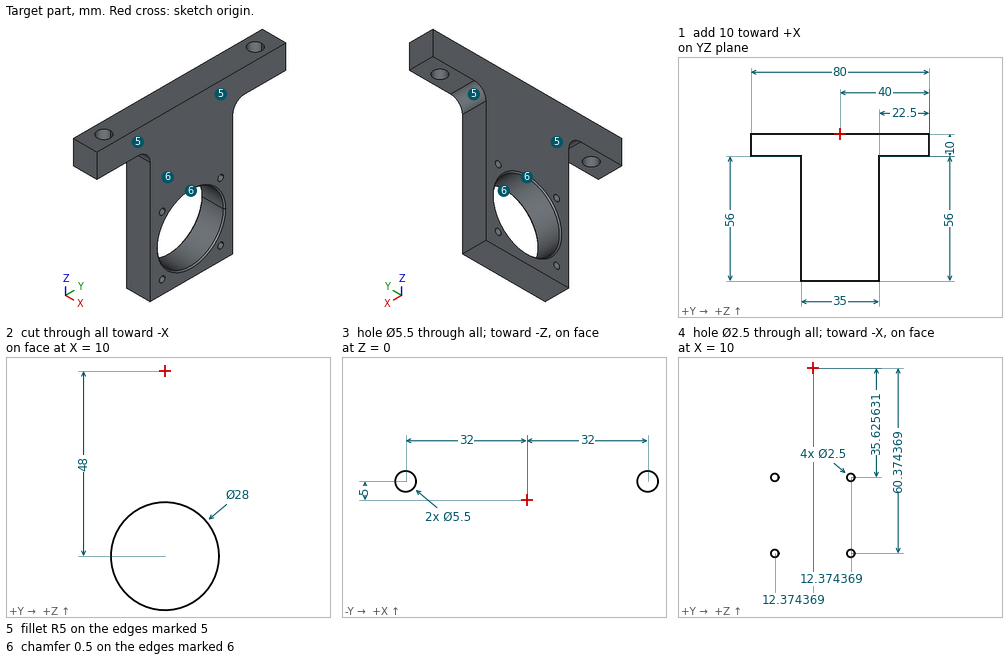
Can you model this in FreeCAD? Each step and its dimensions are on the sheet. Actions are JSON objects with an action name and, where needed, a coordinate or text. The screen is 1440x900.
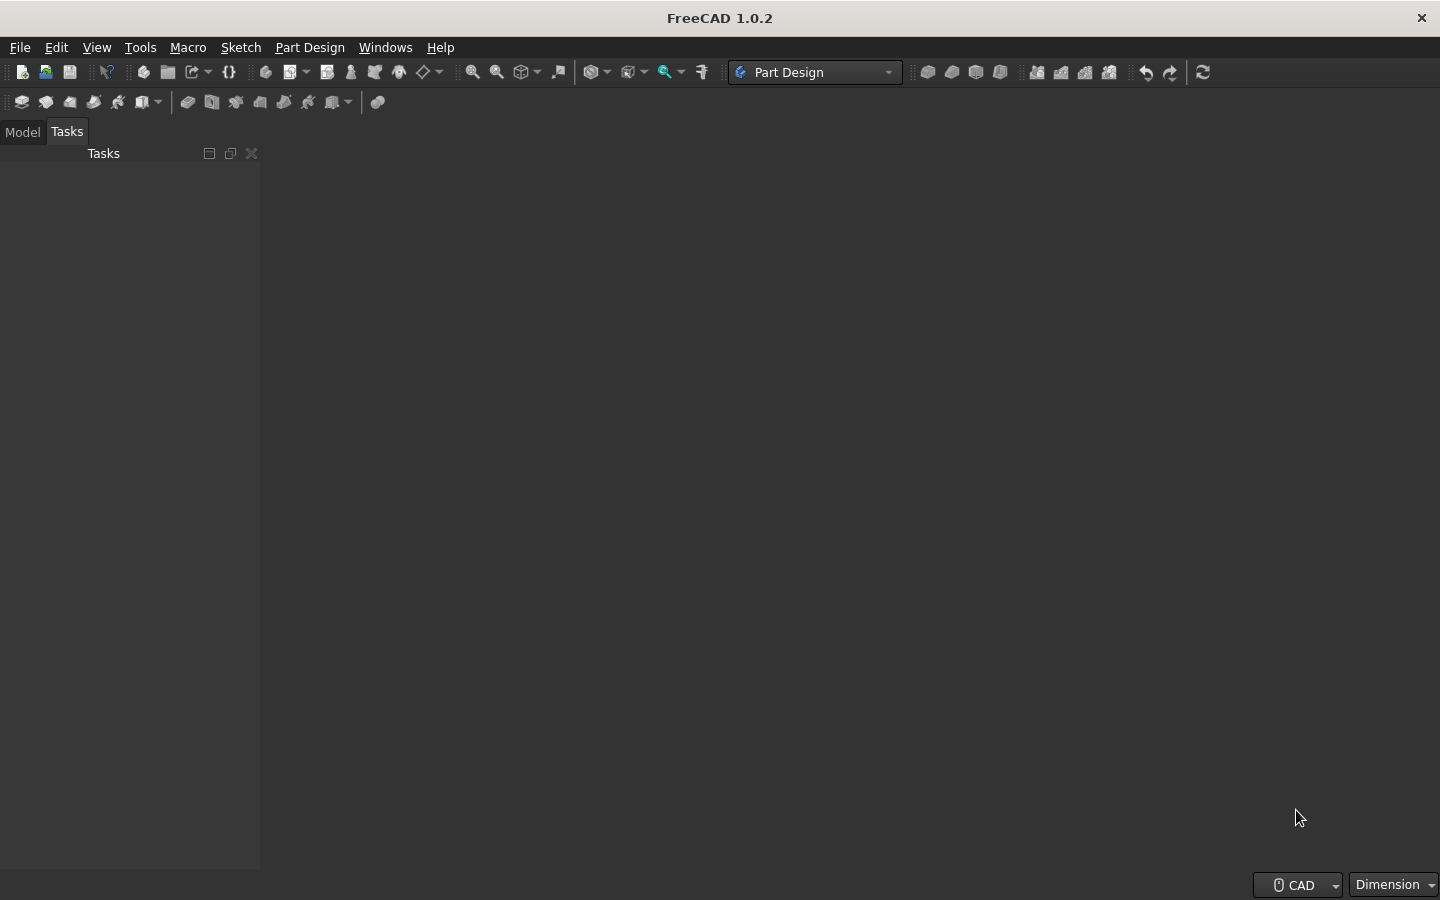
{"action": "left_click", "coordinate": [22, 72]}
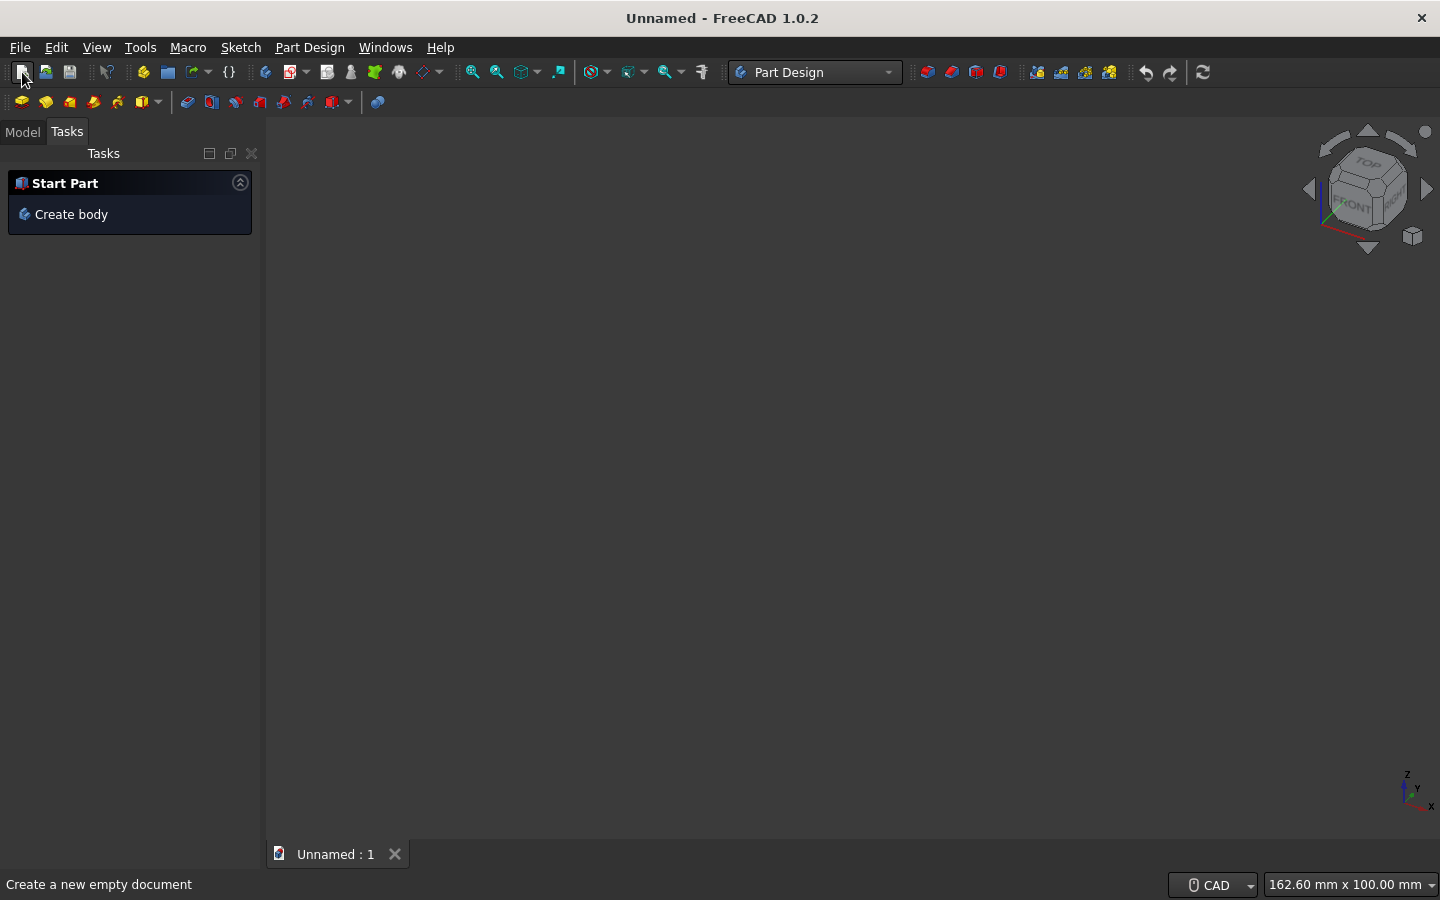
{"action": "left_click", "coordinate": [290, 72]}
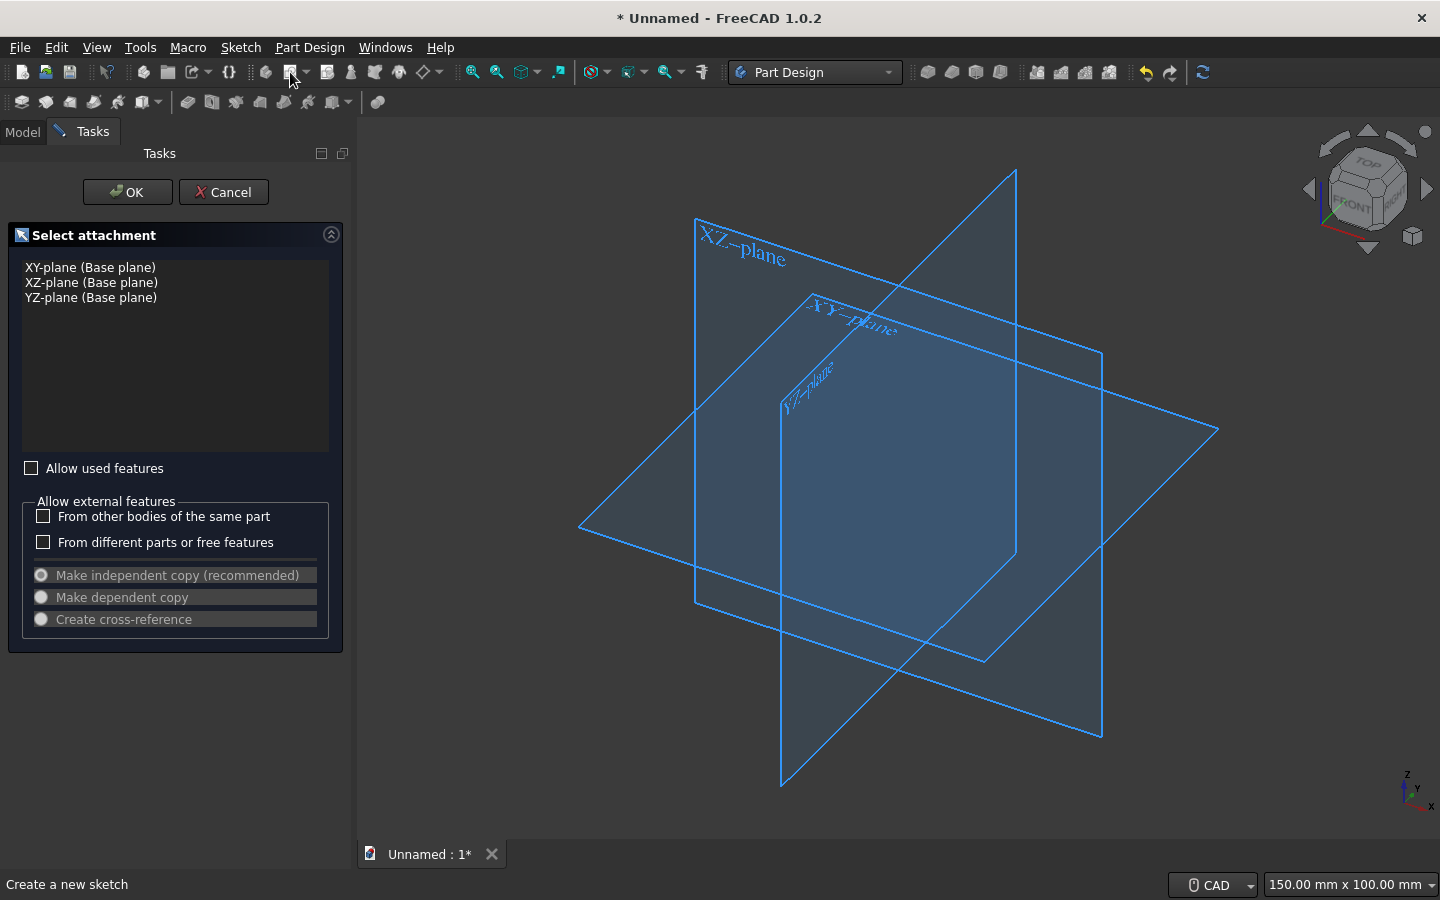
{"action": "left_click", "coordinate": [82, 298]}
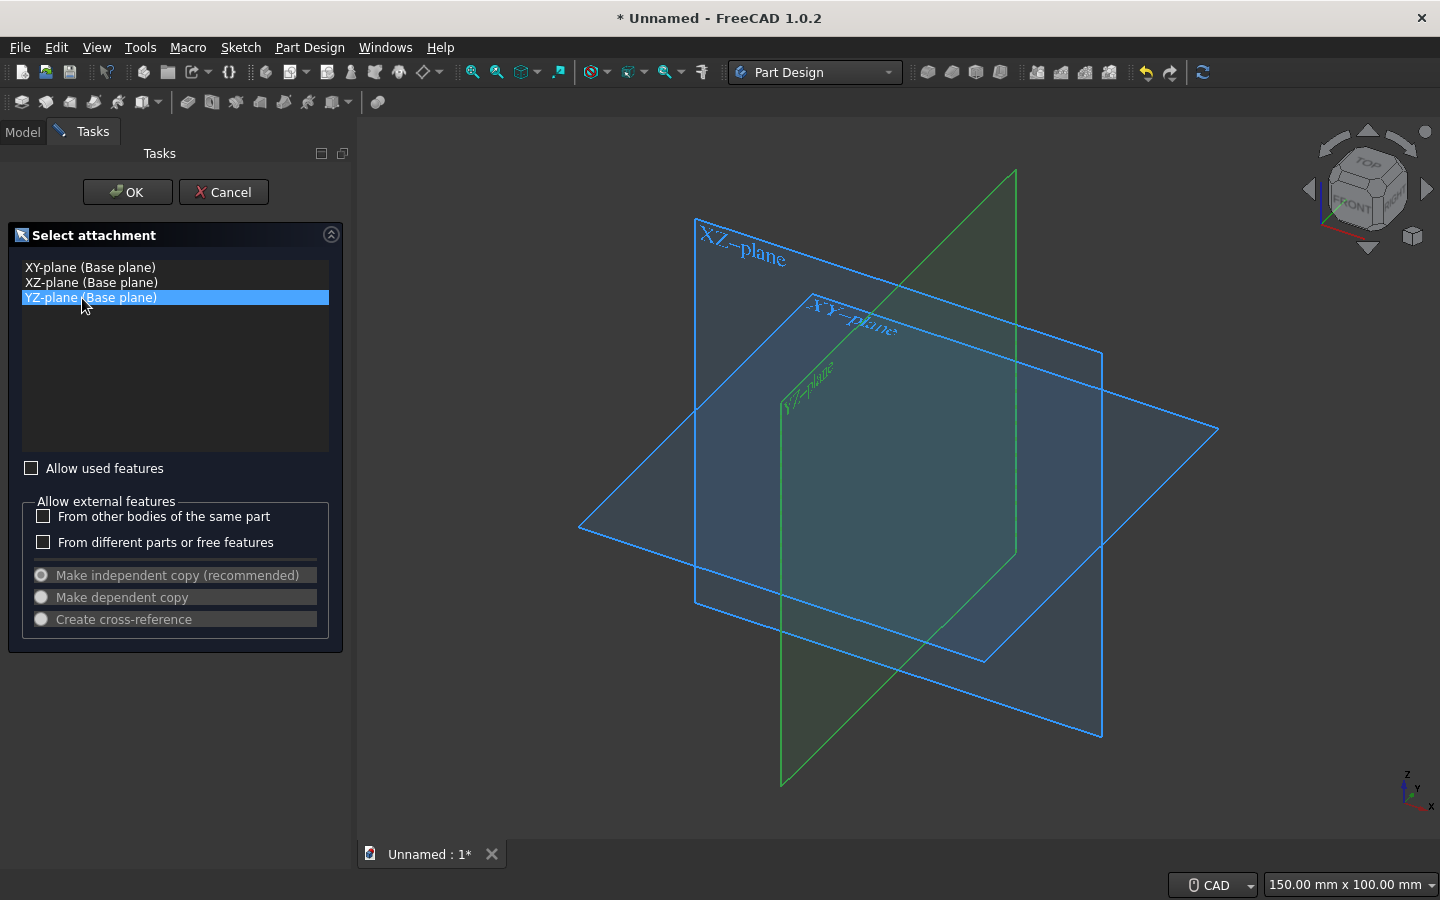
{"action": "left_click", "coordinate": [128, 192]}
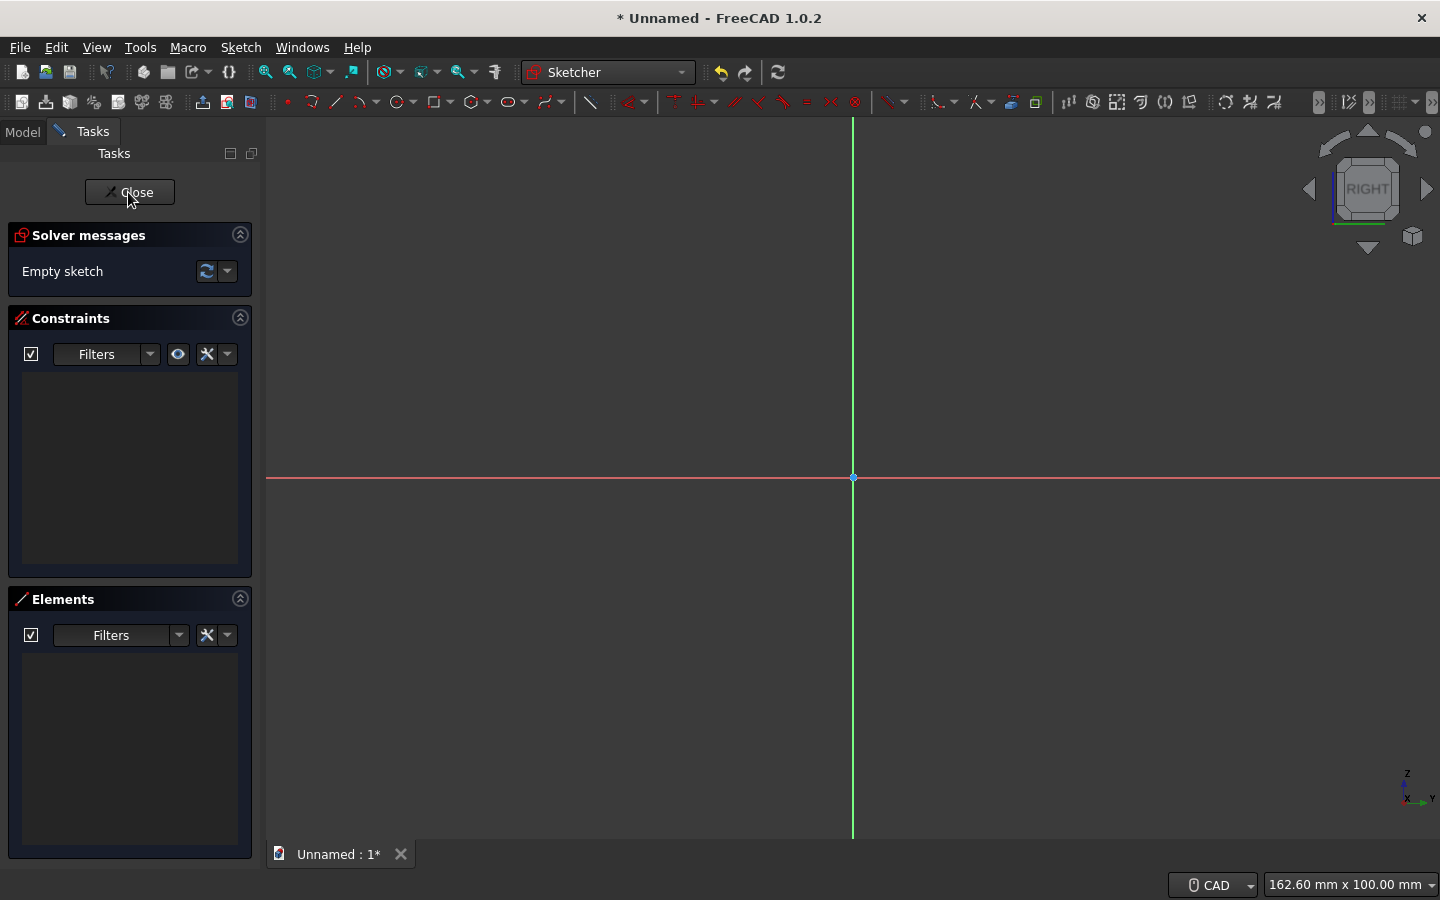
{"action": "scroll", "coordinate": [645, 145], "scroll_direction": "down", "scroll_amount": 2}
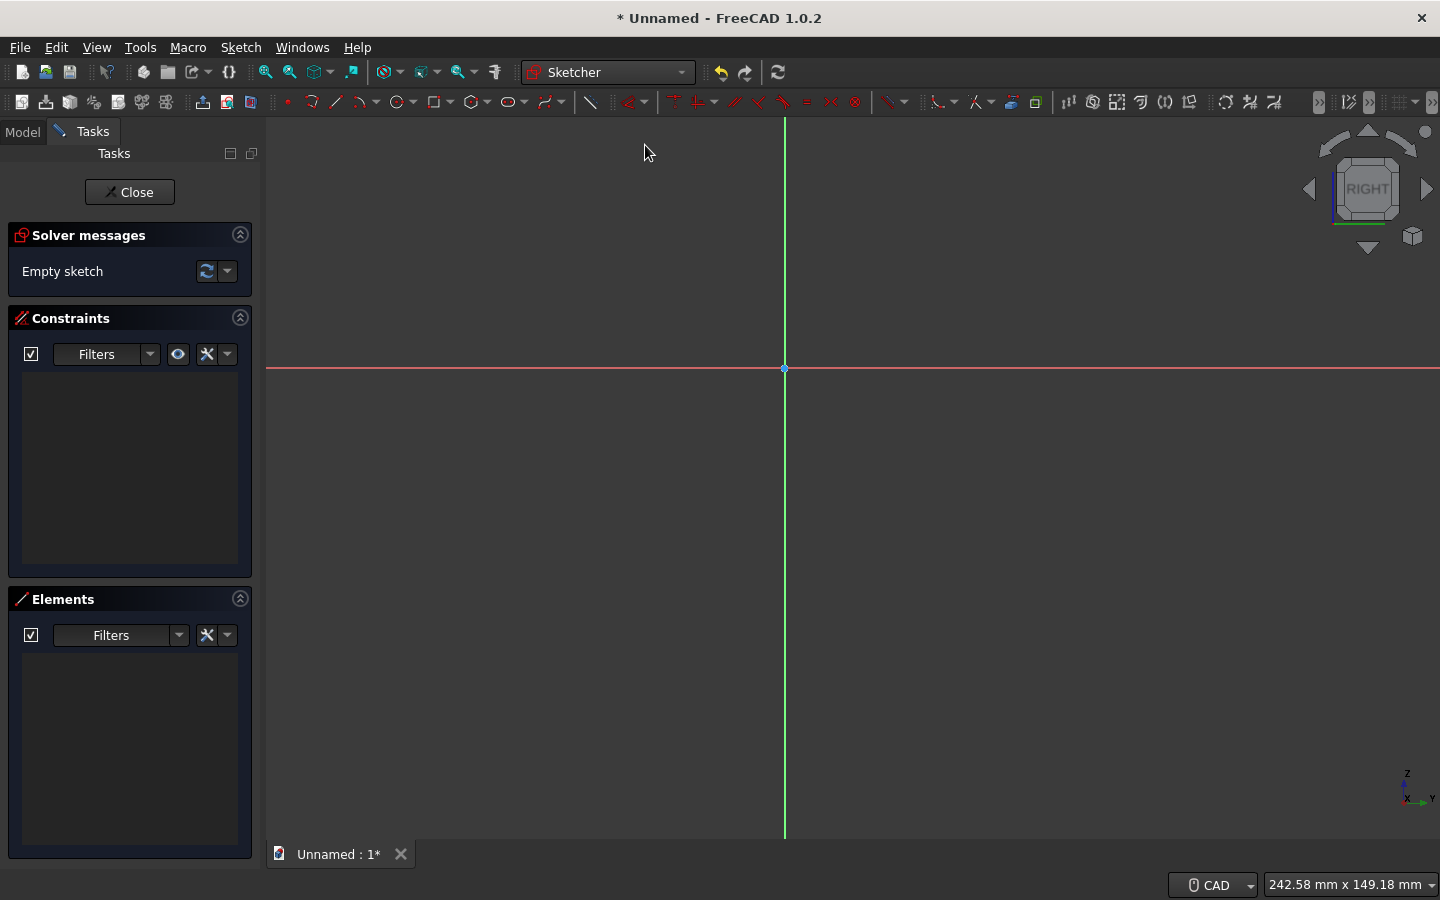
{"action": "scroll", "coordinate": [785, 629], "scroll_direction": "up", "scroll_amount": 2}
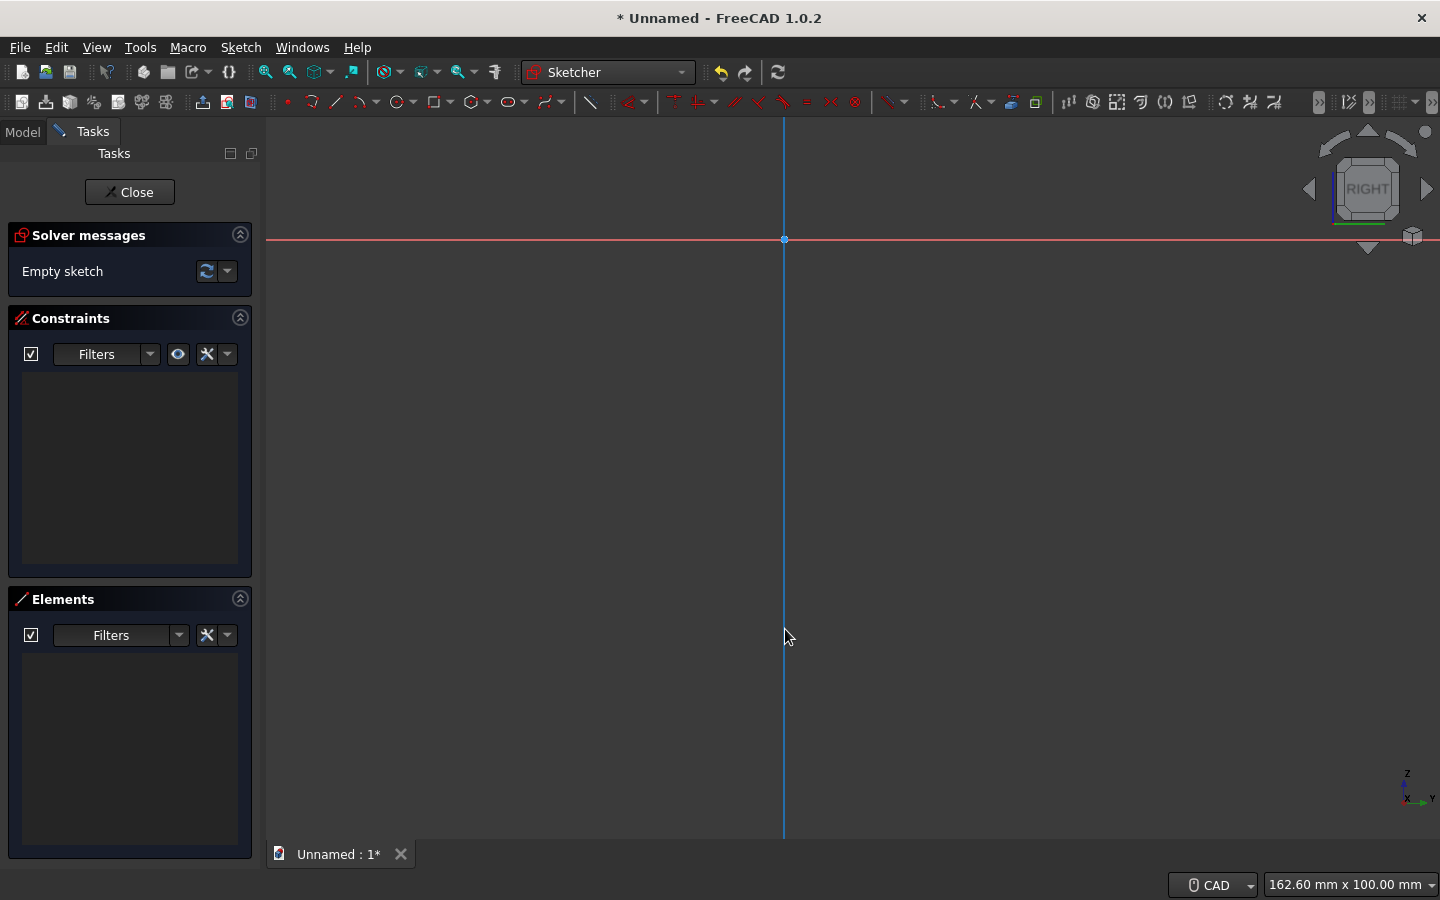
{"action": "left_click", "coordinate": [312, 102]}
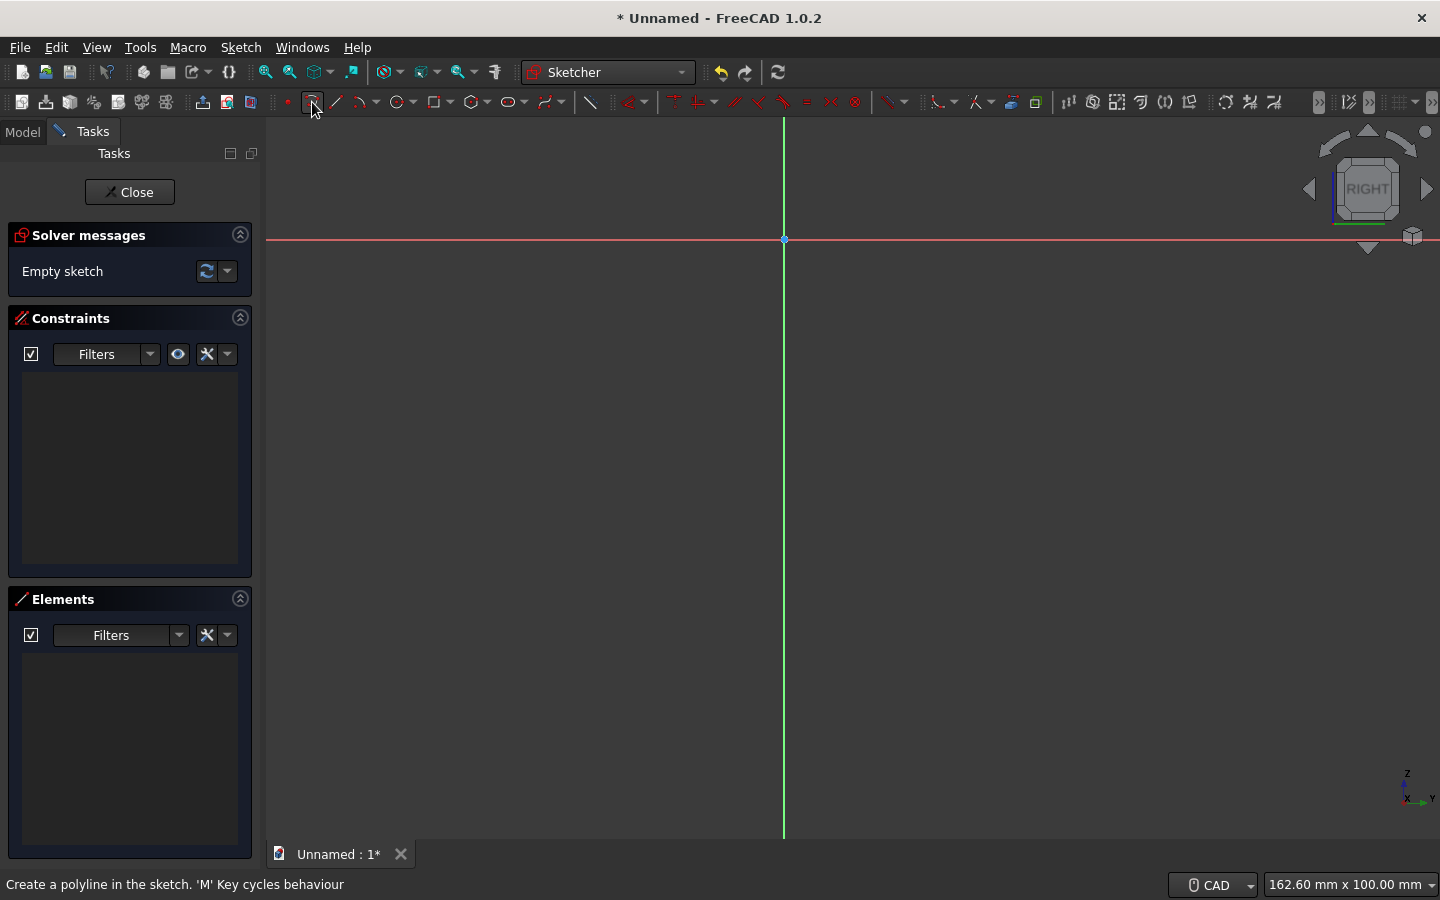
{"action": "left_click", "coordinate": [658, 312]}
{"action": "left_click", "coordinate": [658, 716]}
{"action": "left_click", "coordinate": [910, 716]}
{"action": "left_click", "coordinate": [910, 312]}
{"action": "left_click", "coordinate": [1073, 312]}
{"action": "left_click", "coordinate": [1073, 240]}
{"action": "left_click", "coordinate": [495, 249]}
{"action": "left_click", "coordinate": [495, 312]}
{"action": "left_click", "coordinate": [658, 313]}
{"action": "key", "text": "Escape"}
{"action": "key", "text": "Escape"}